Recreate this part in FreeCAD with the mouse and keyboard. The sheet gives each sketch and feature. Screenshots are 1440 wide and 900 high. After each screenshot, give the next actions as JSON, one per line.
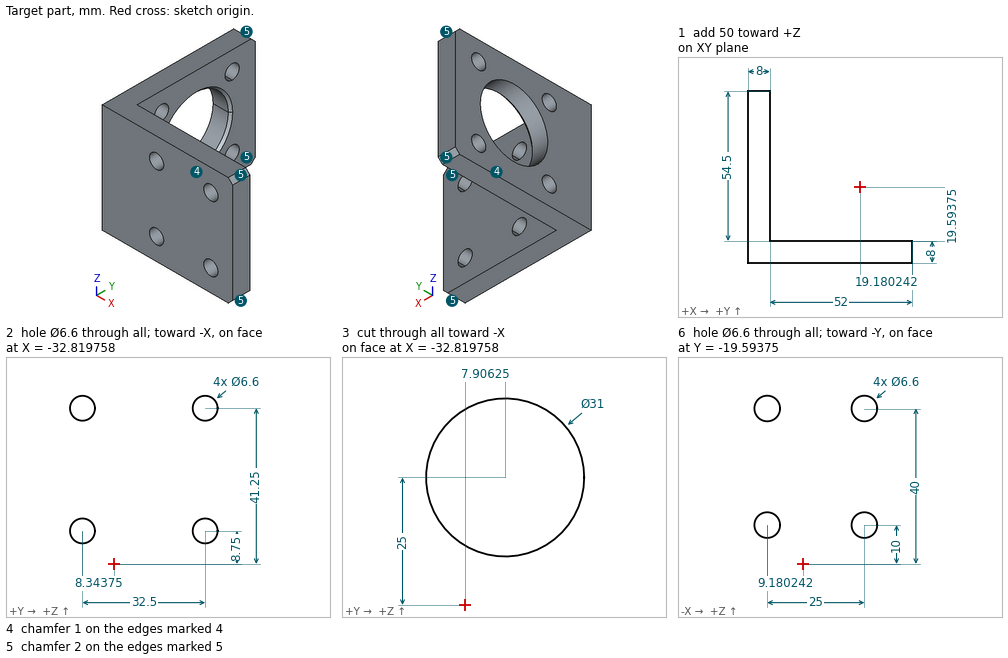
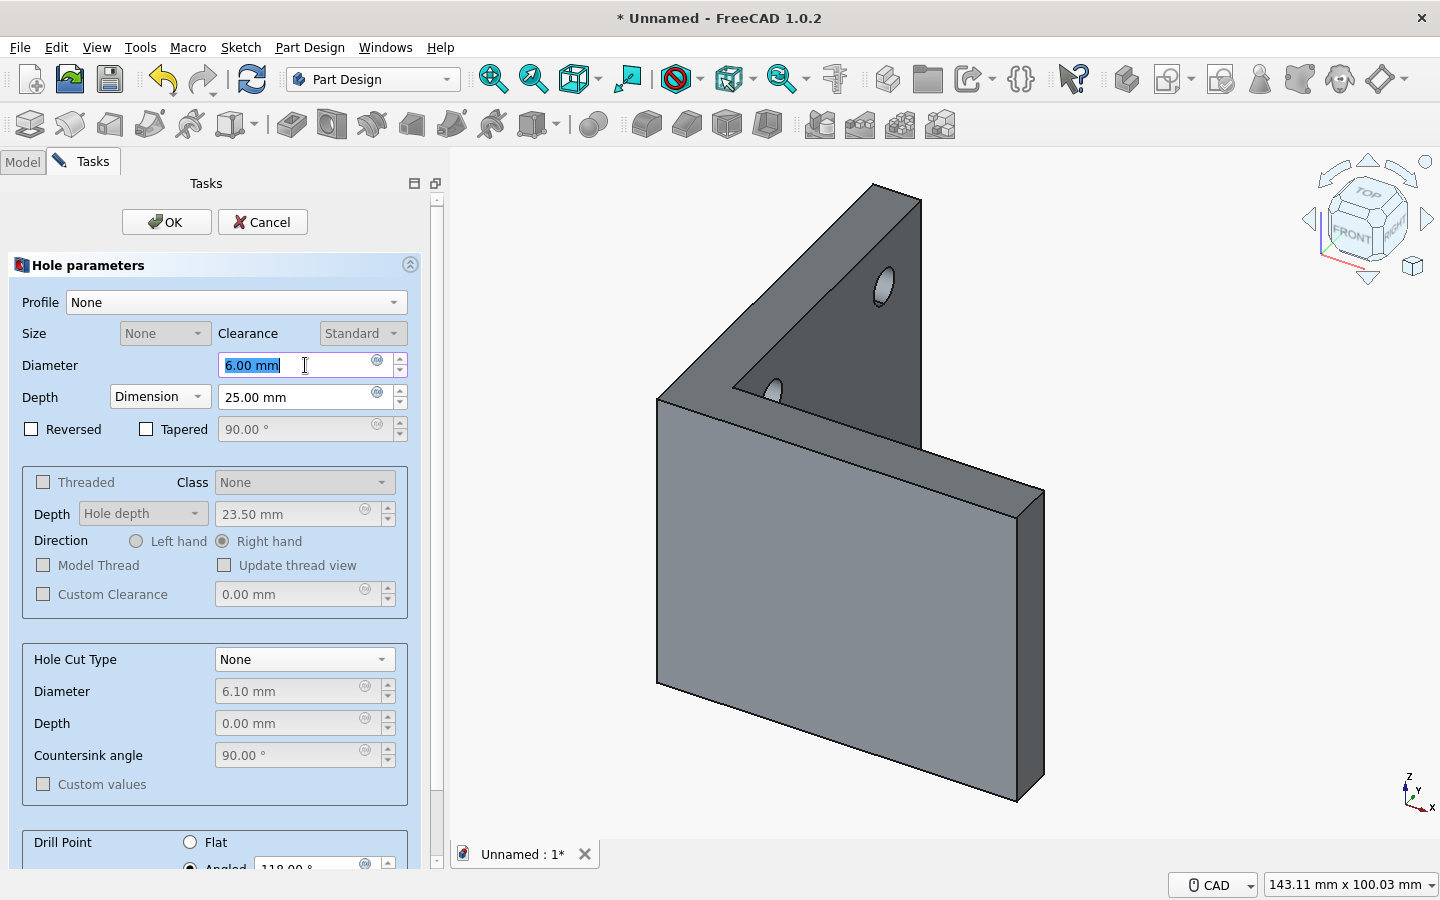
{"action": "type", "text": "6.6"}
{"action": "key", "text": "Tab"}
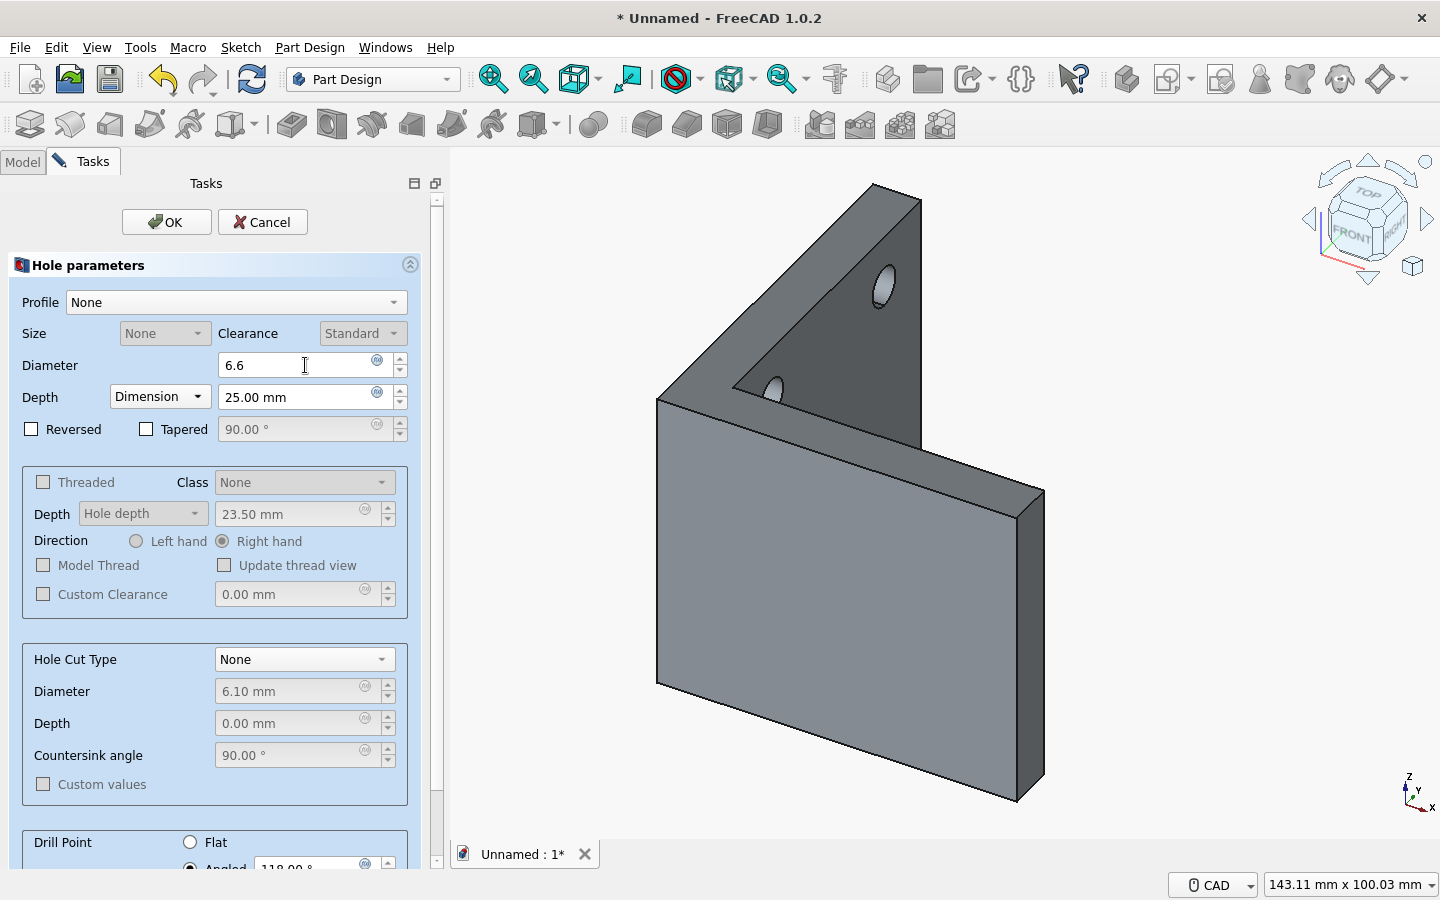
{"action": "left_click", "coordinate": [161, 396]}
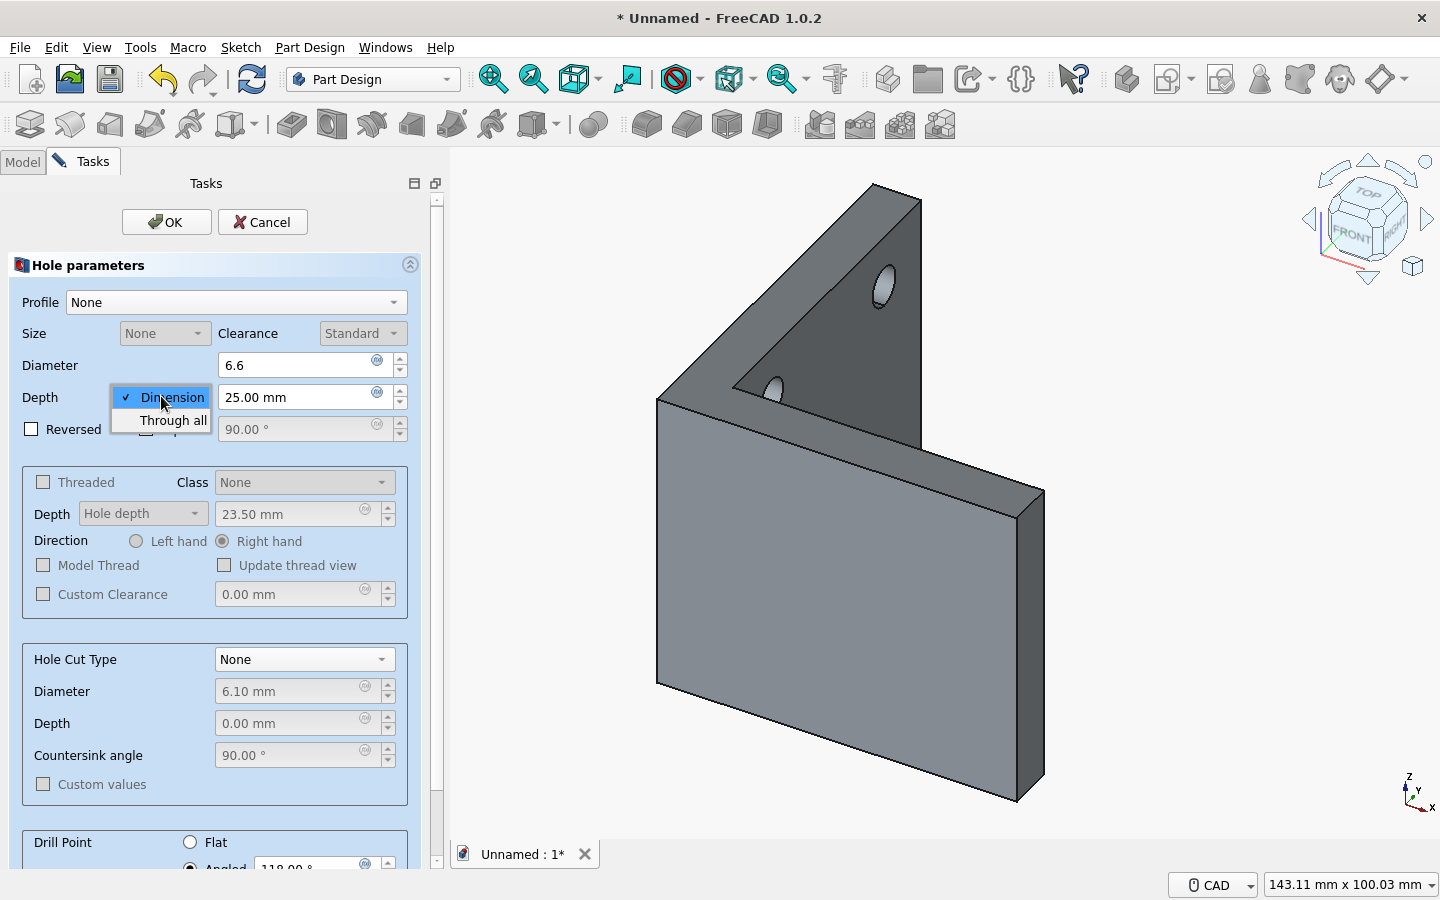
{"action": "left_click", "coordinate": [160, 420]}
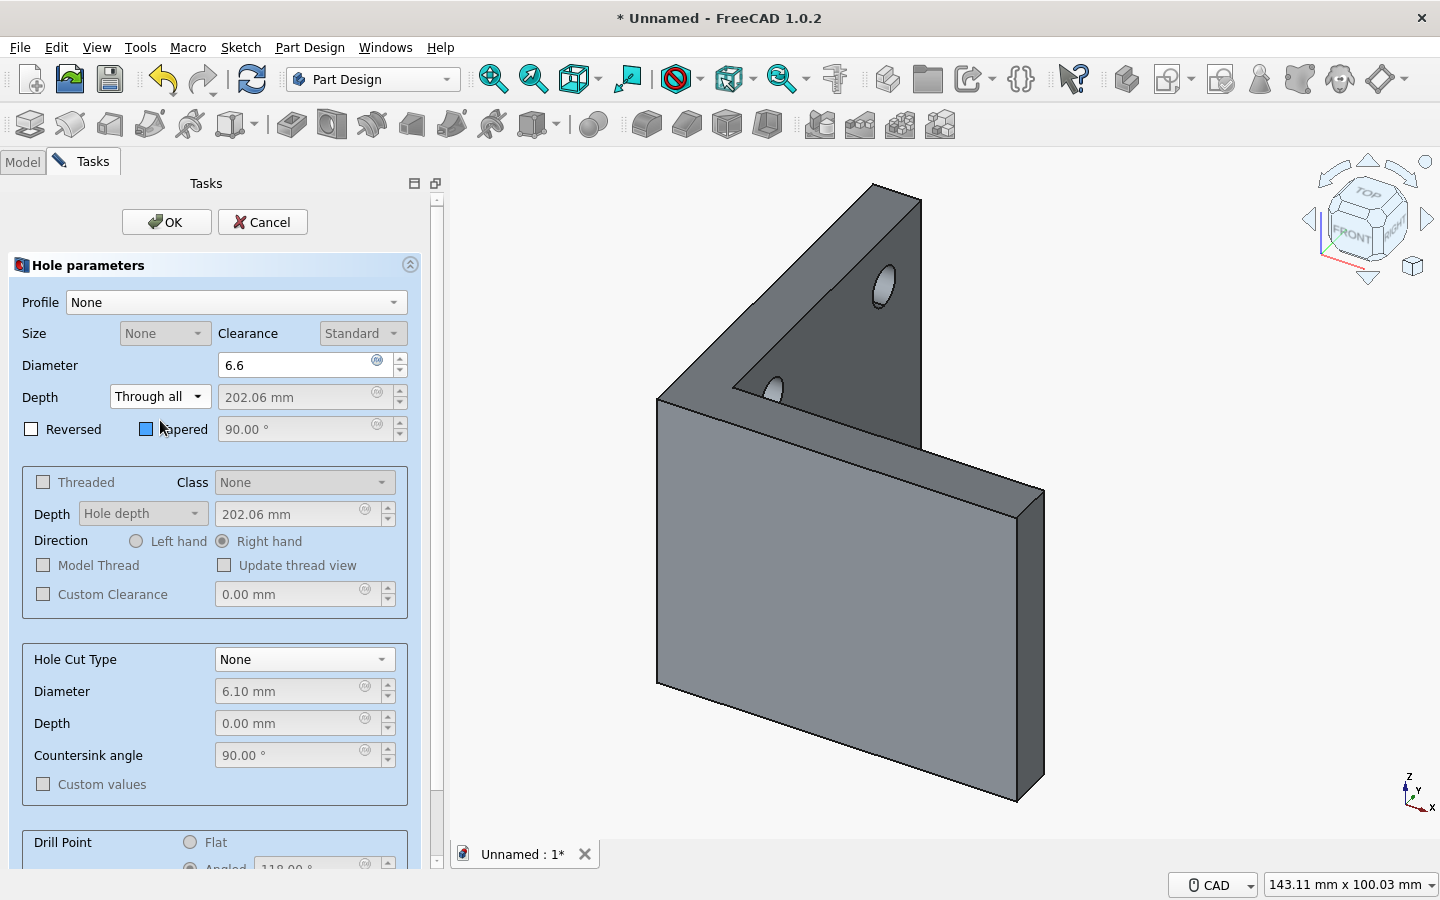
{"action": "left_click", "coordinate": [167, 222]}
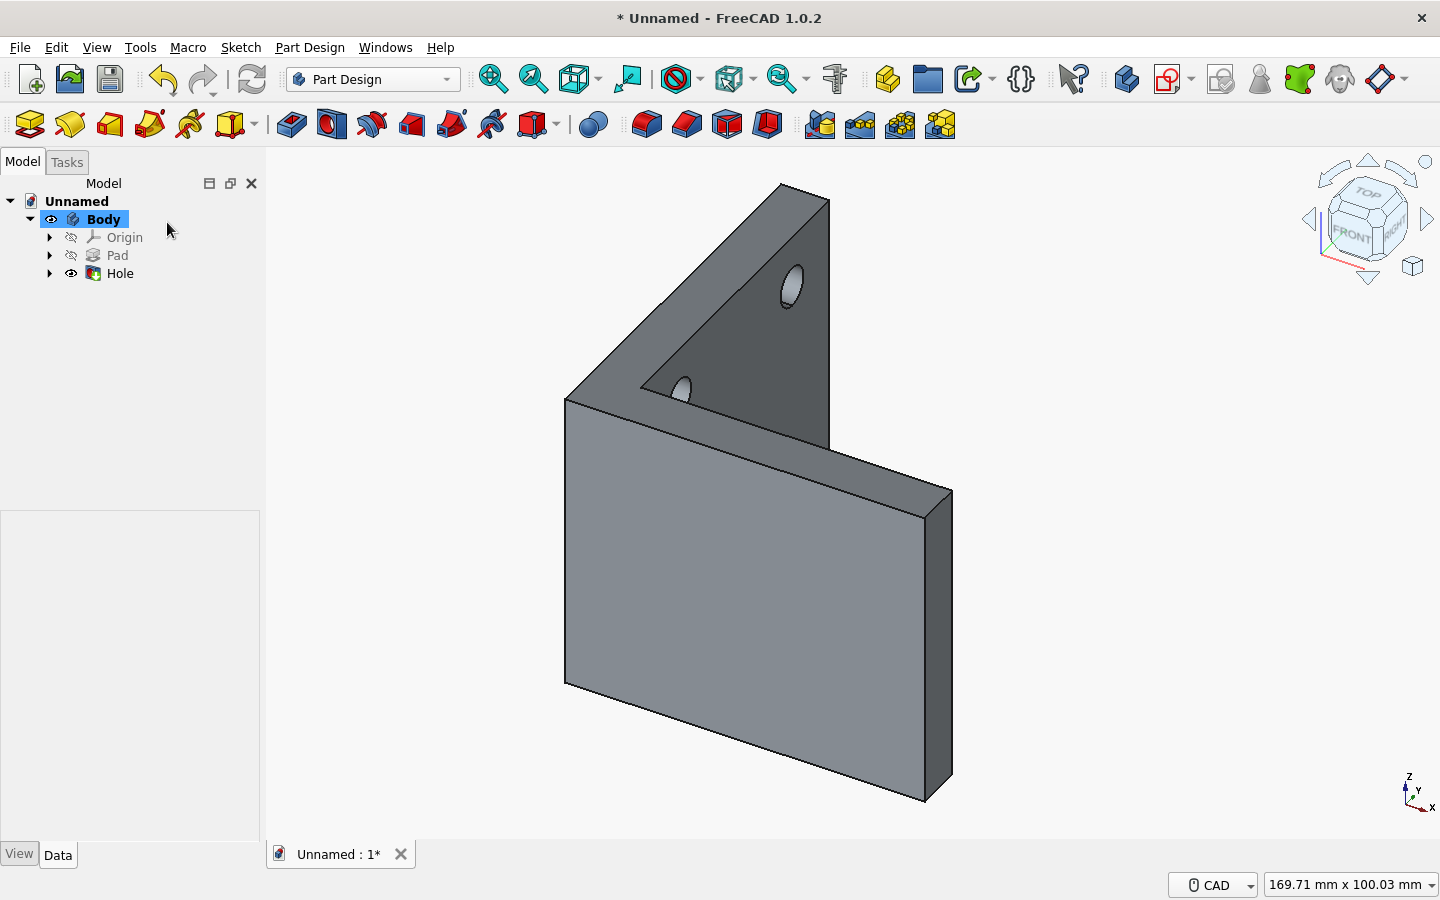
{"action": "left_click", "coordinate": [762, 408]}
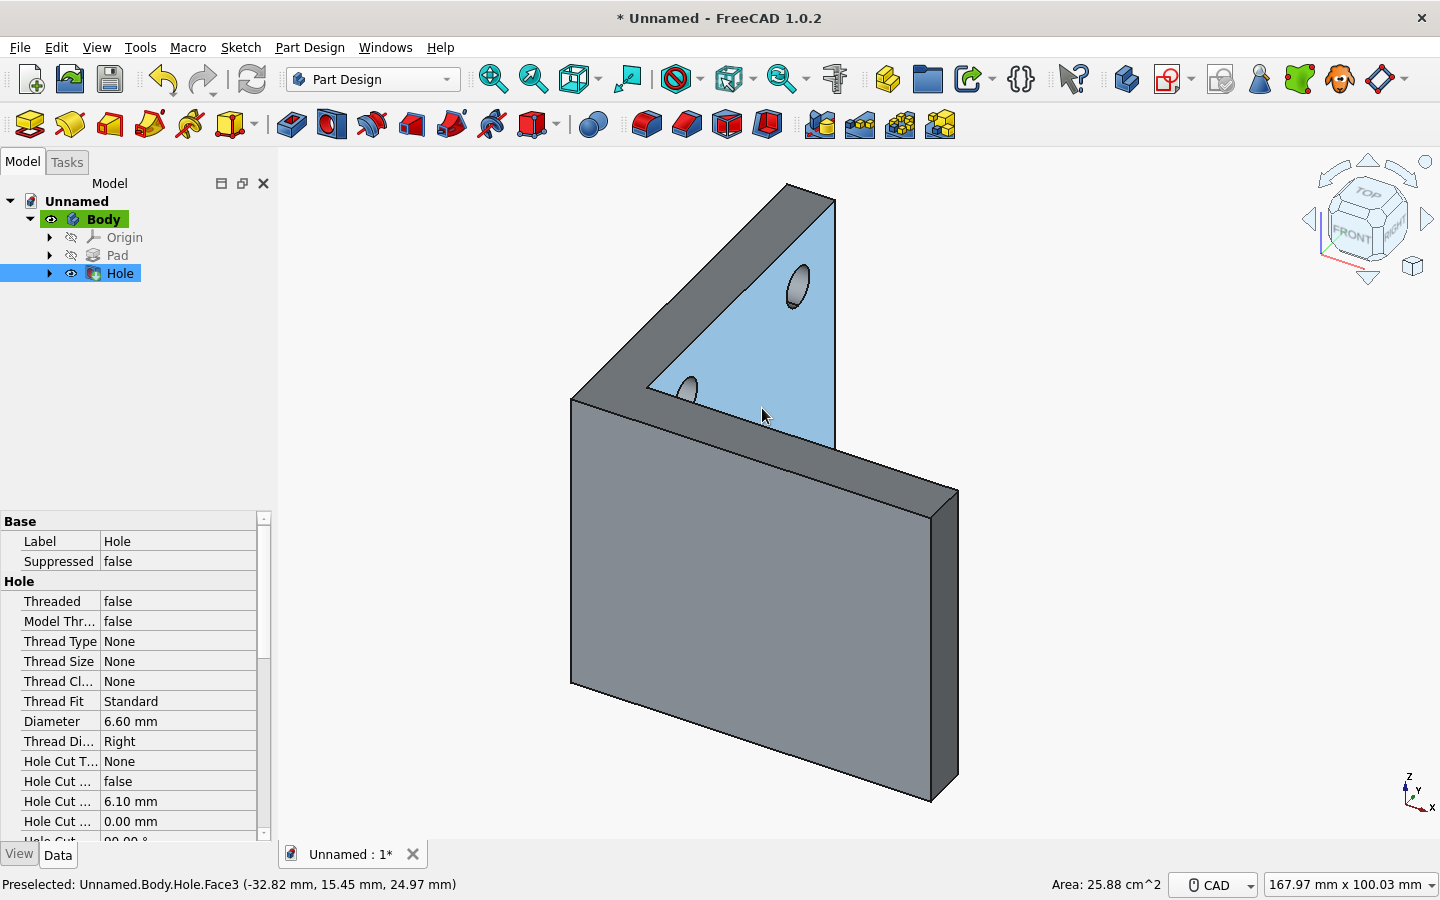
{"action": "left_click", "coordinate": [1168, 80]}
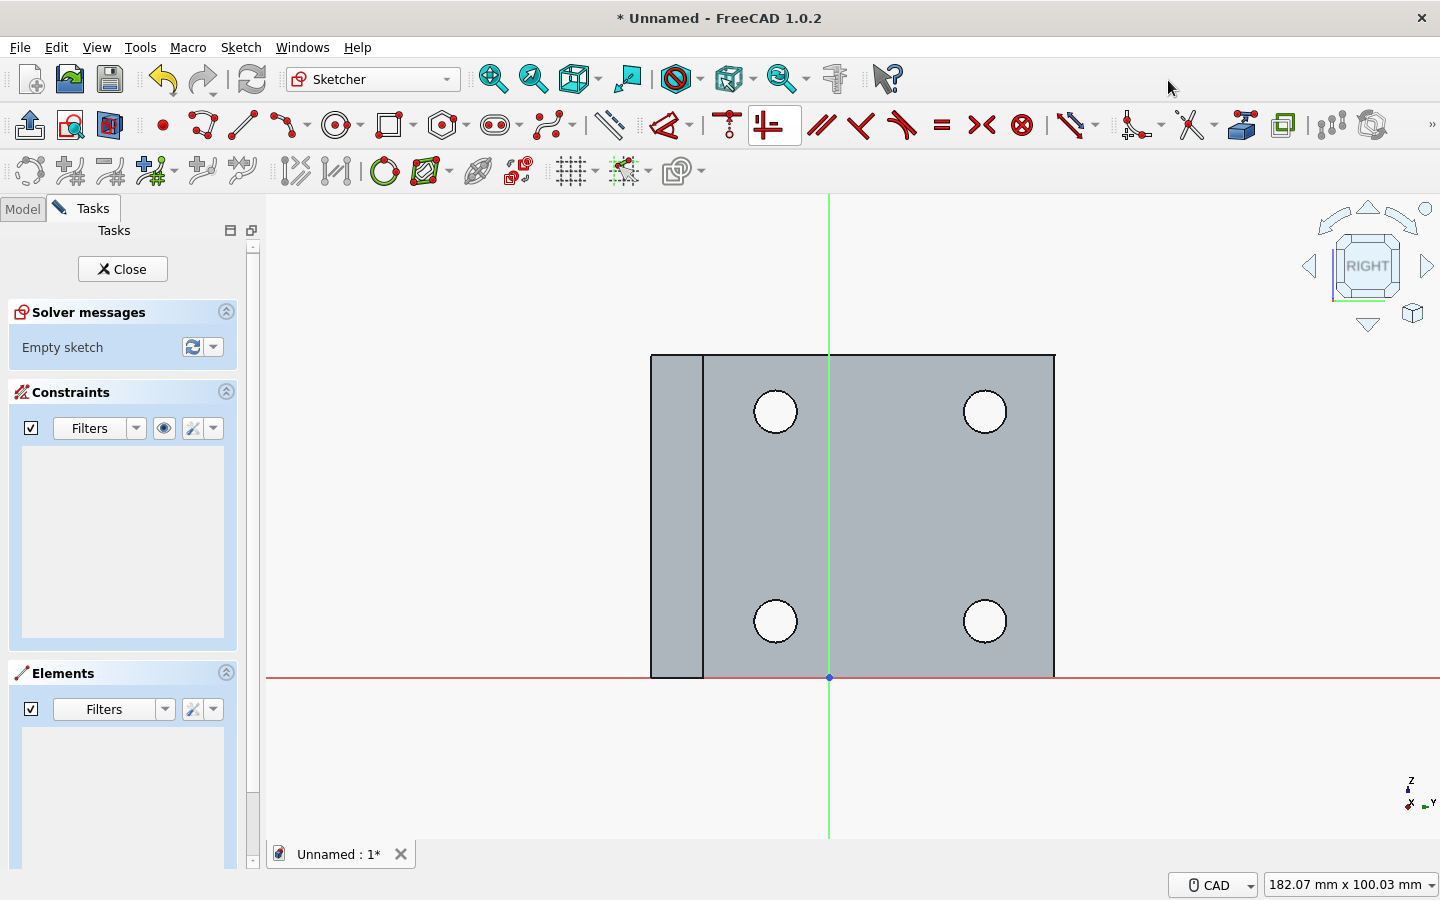
{"action": "scroll", "coordinate": [1075, 609], "scroll_direction": "up", "scroll_amount": 2}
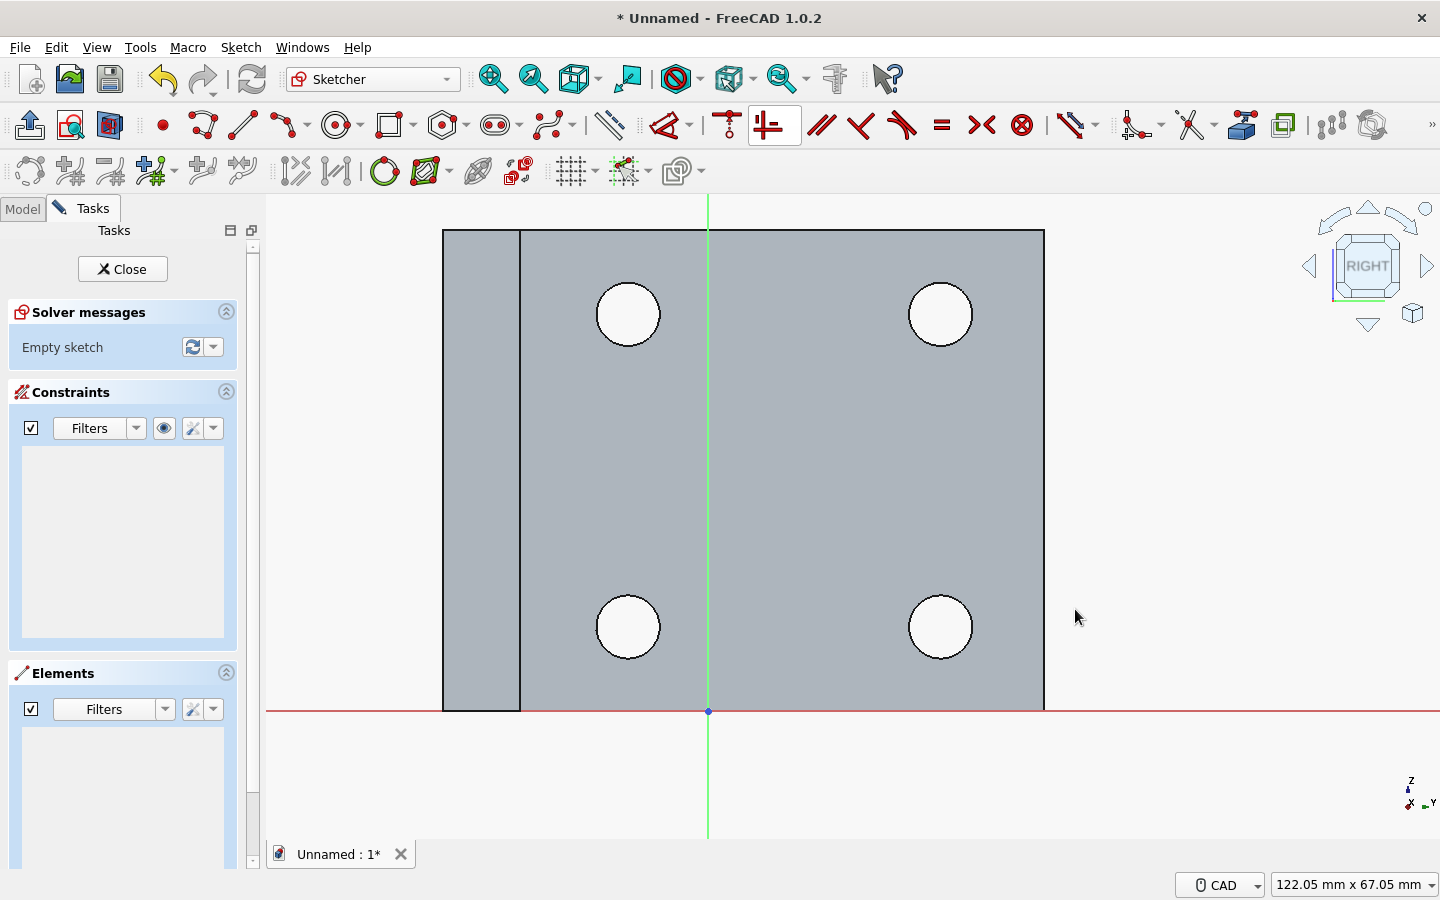
{"action": "left_click", "coordinate": [336, 126]}